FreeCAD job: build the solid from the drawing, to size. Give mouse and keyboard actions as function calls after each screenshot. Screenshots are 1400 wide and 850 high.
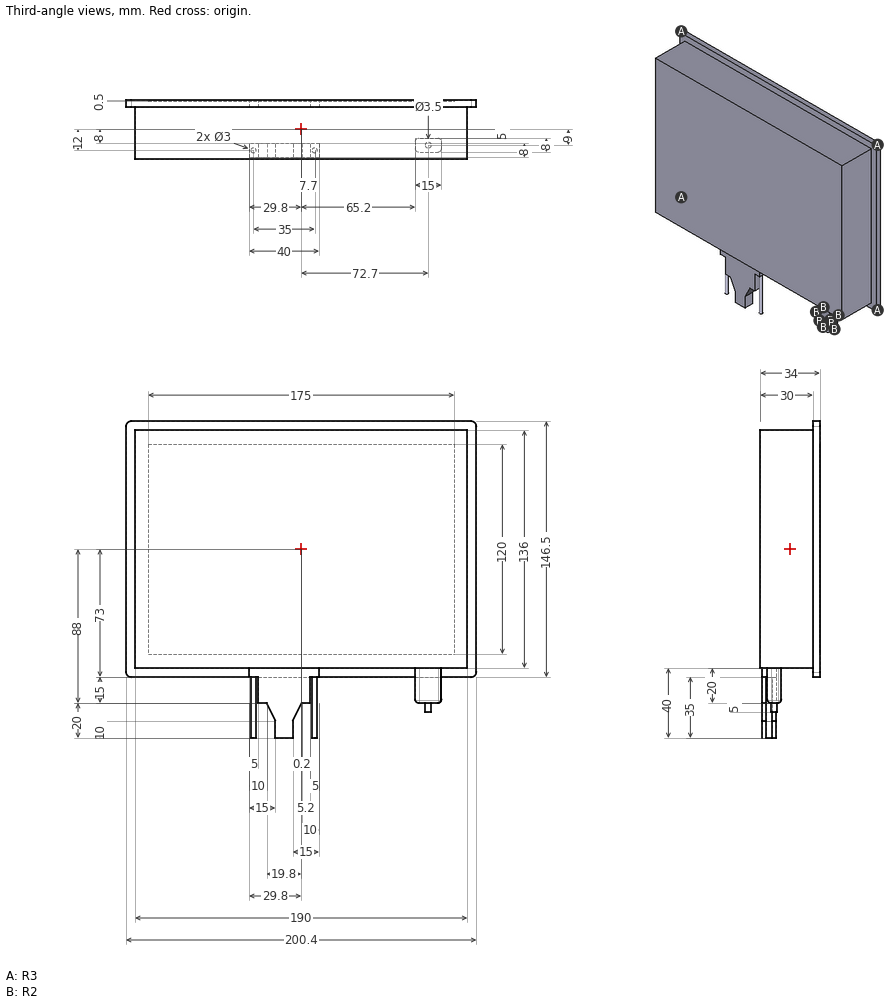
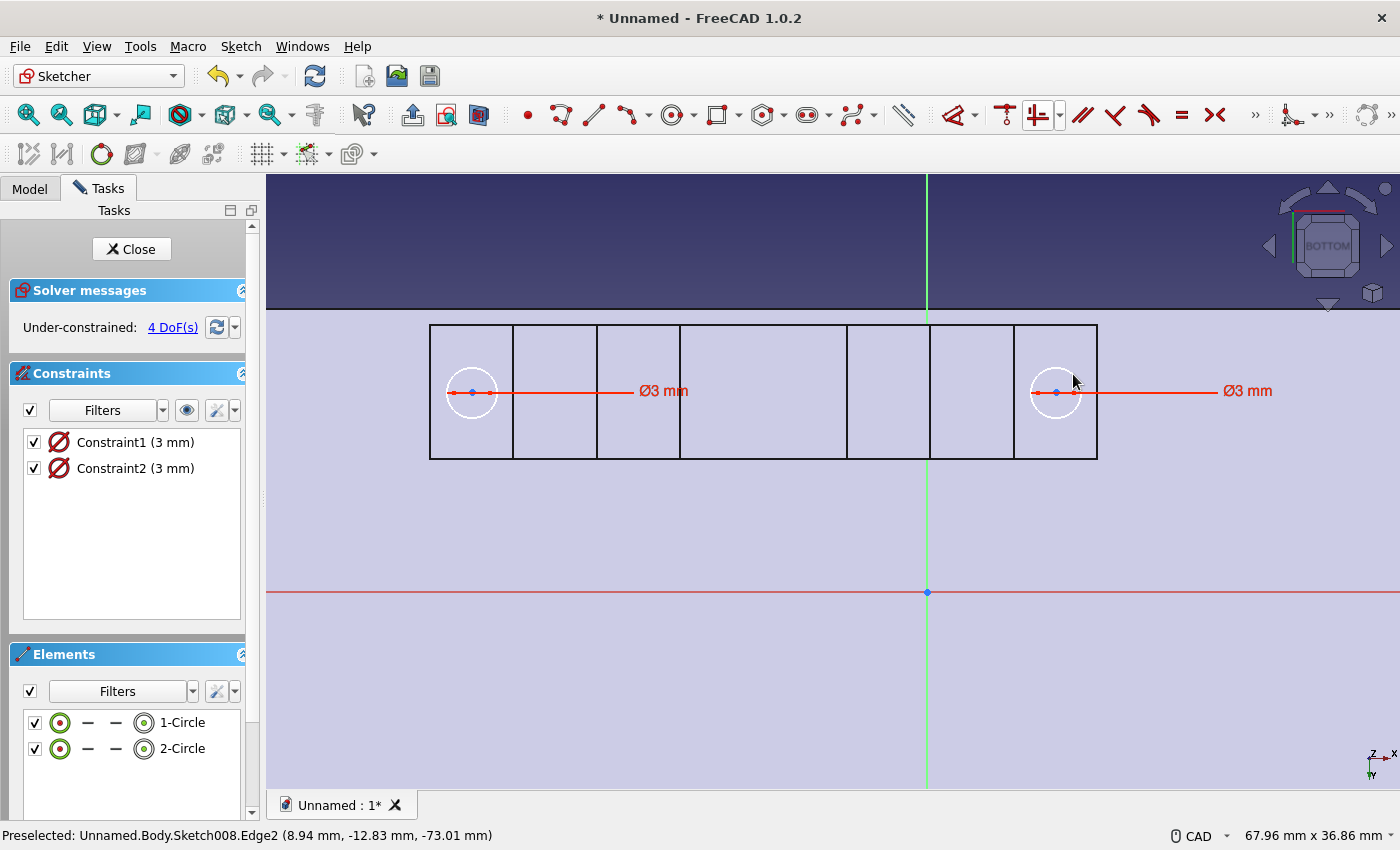
click(952, 116)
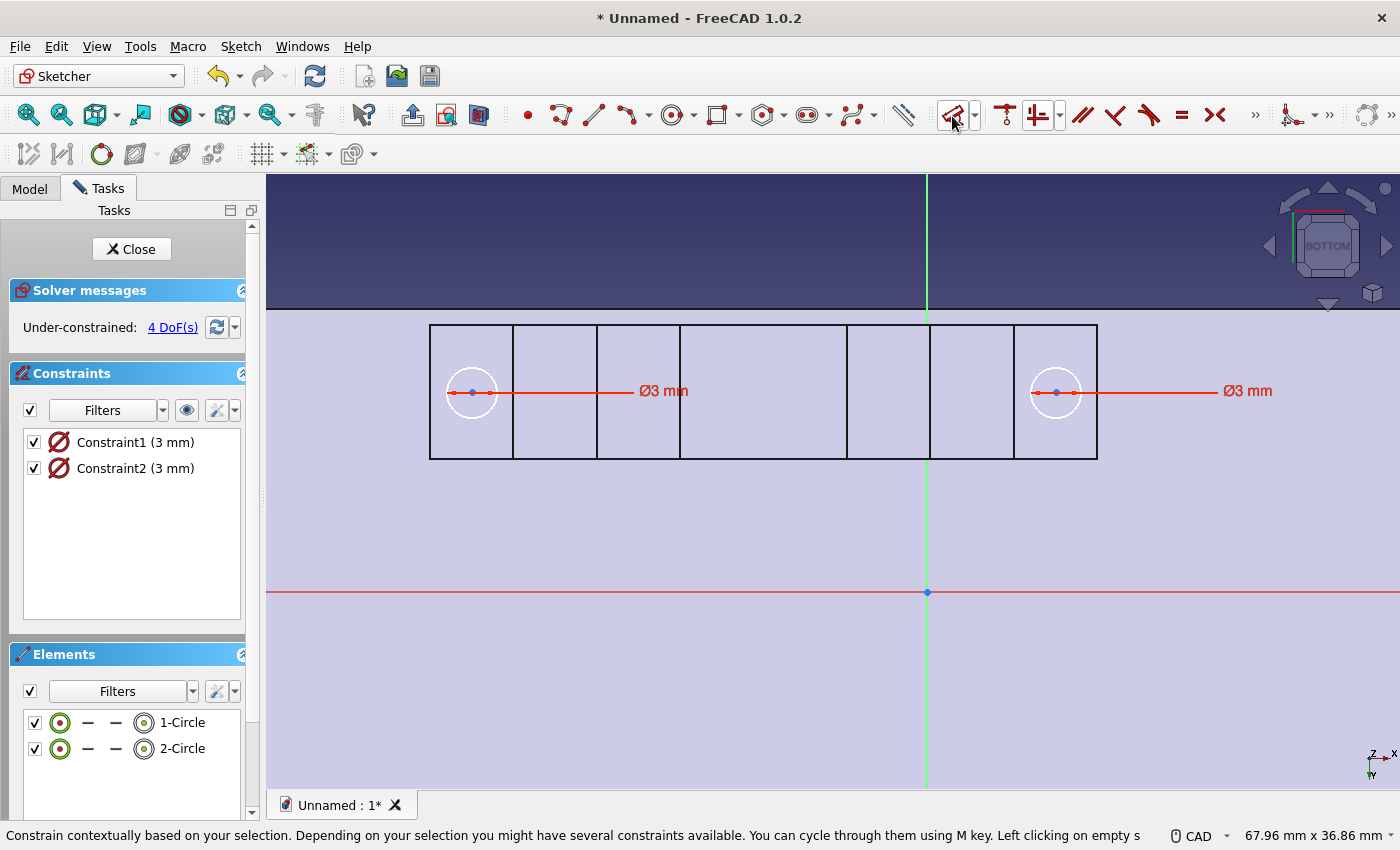
click(472, 393)
click(438, 493)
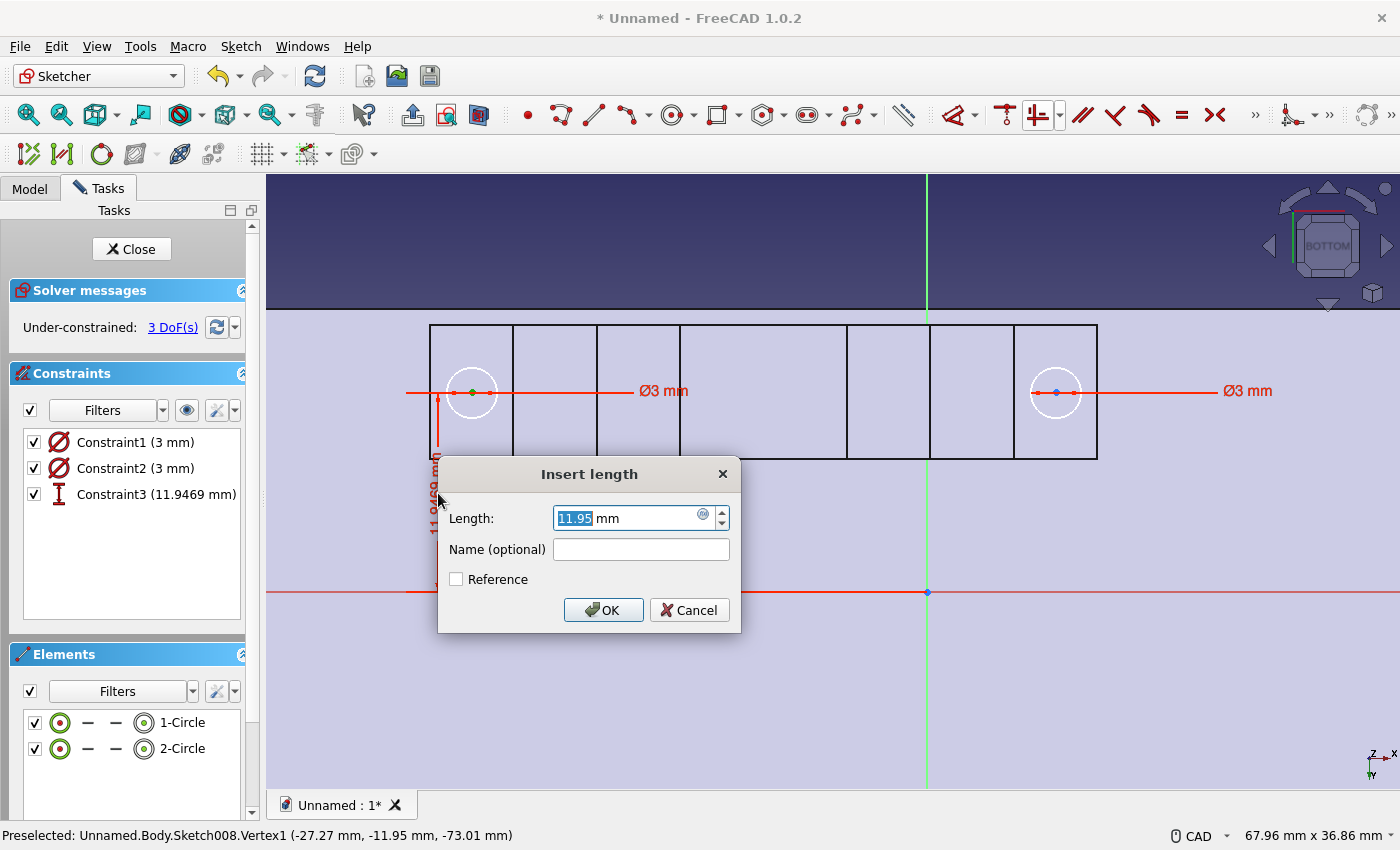
text(12)
key(Return)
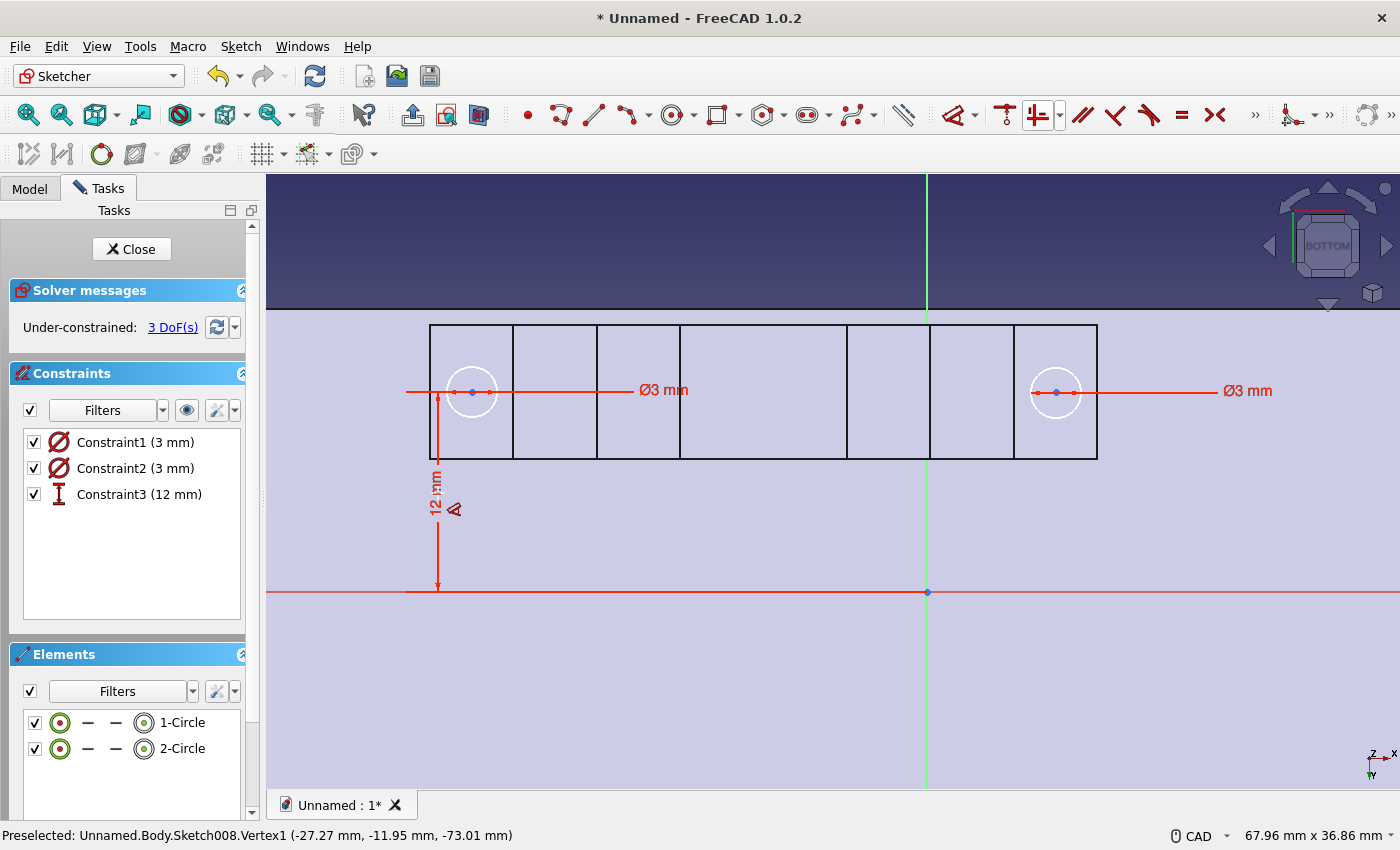
click(1056, 393)
click(1090, 493)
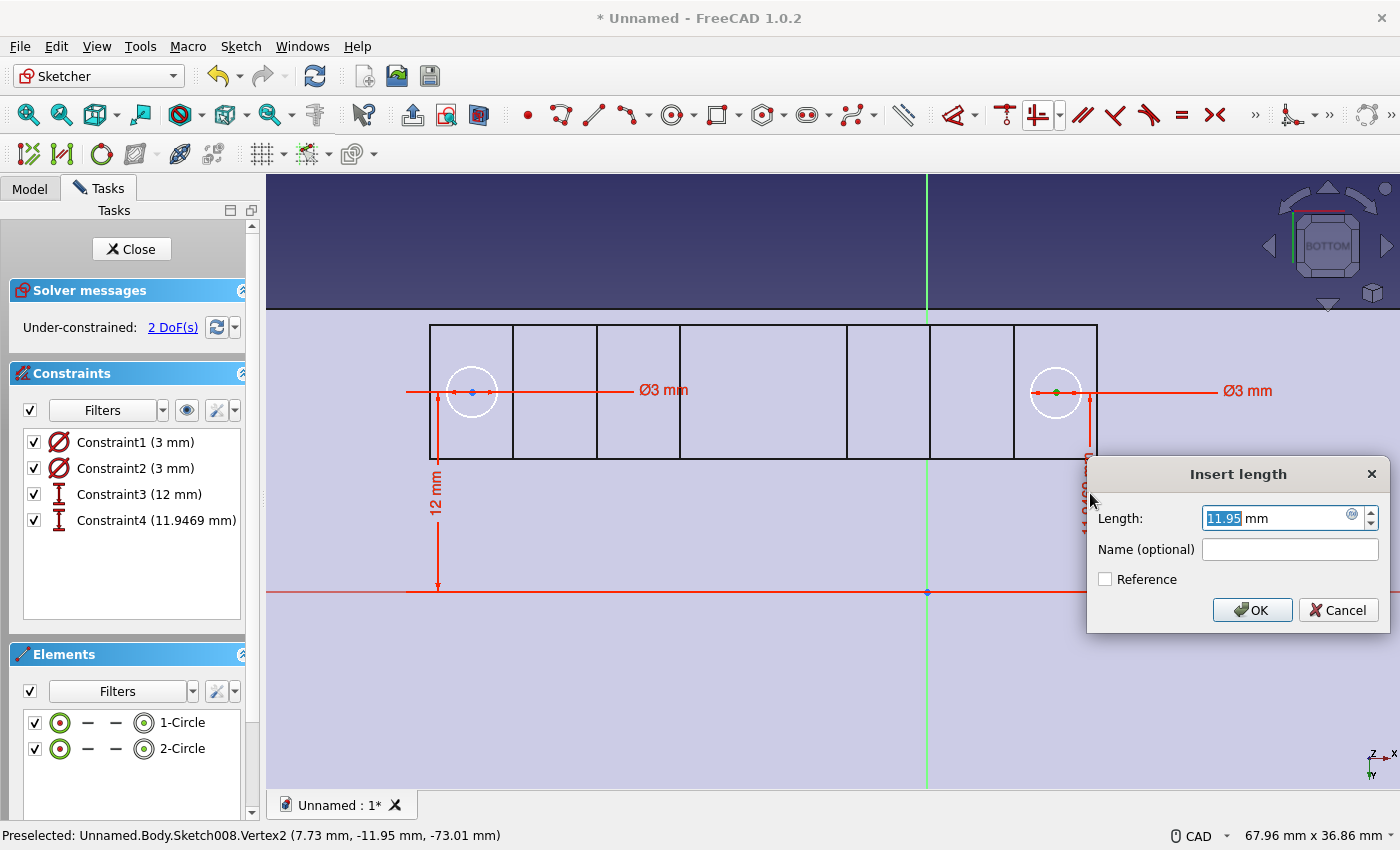
text(12)
key(Return)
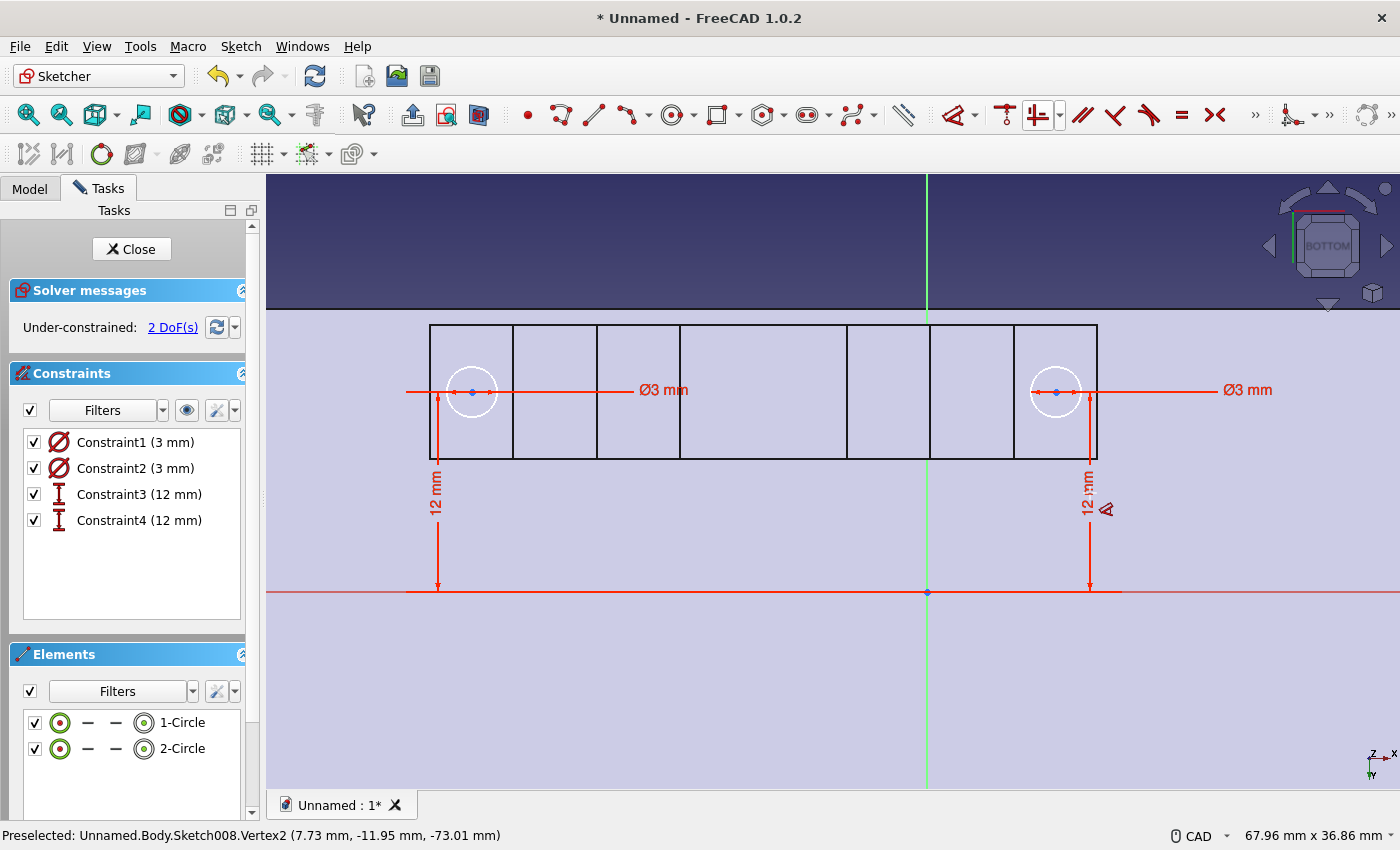
click(1056, 392)
click(992, 626)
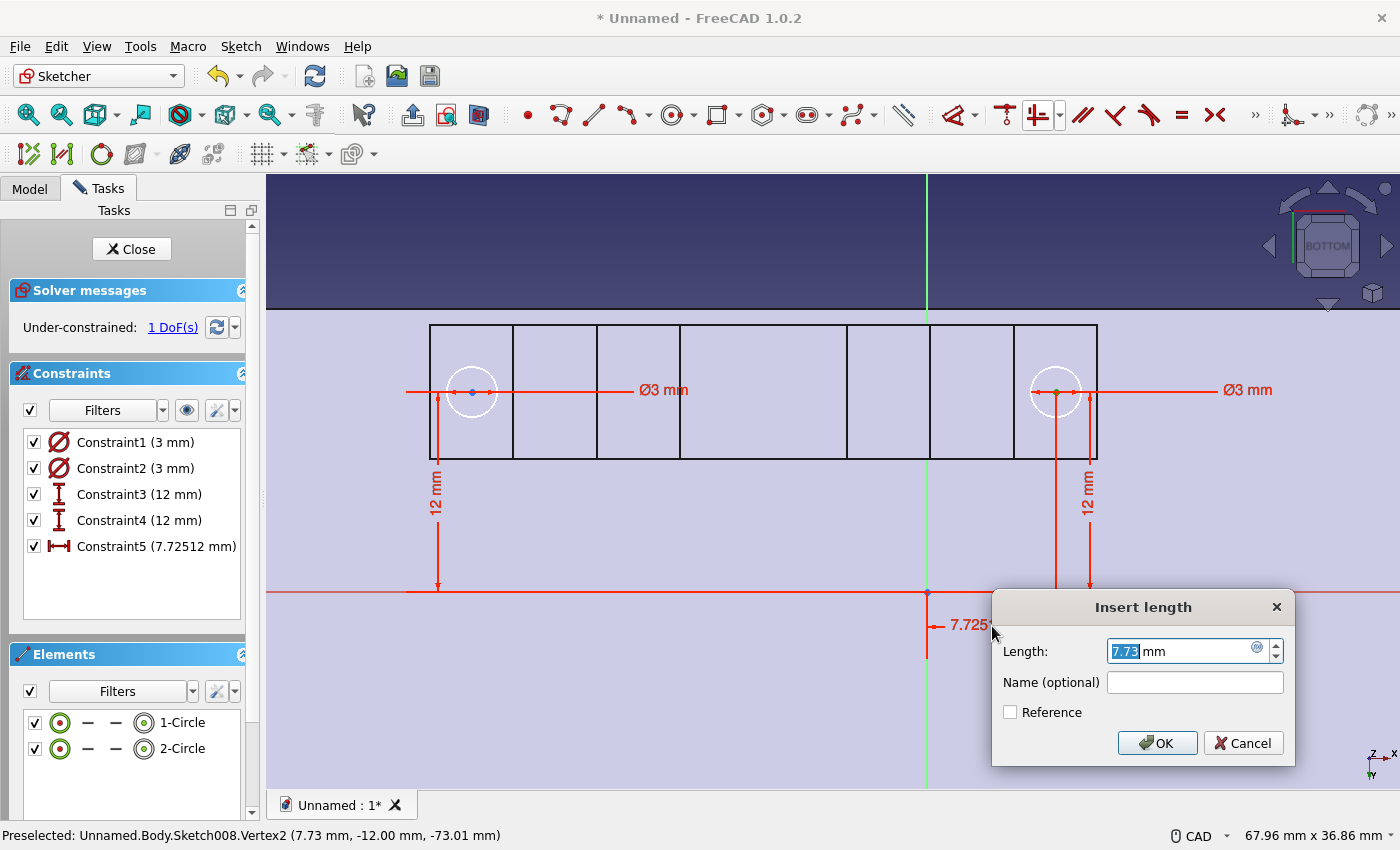
text(7.7)
key(Return)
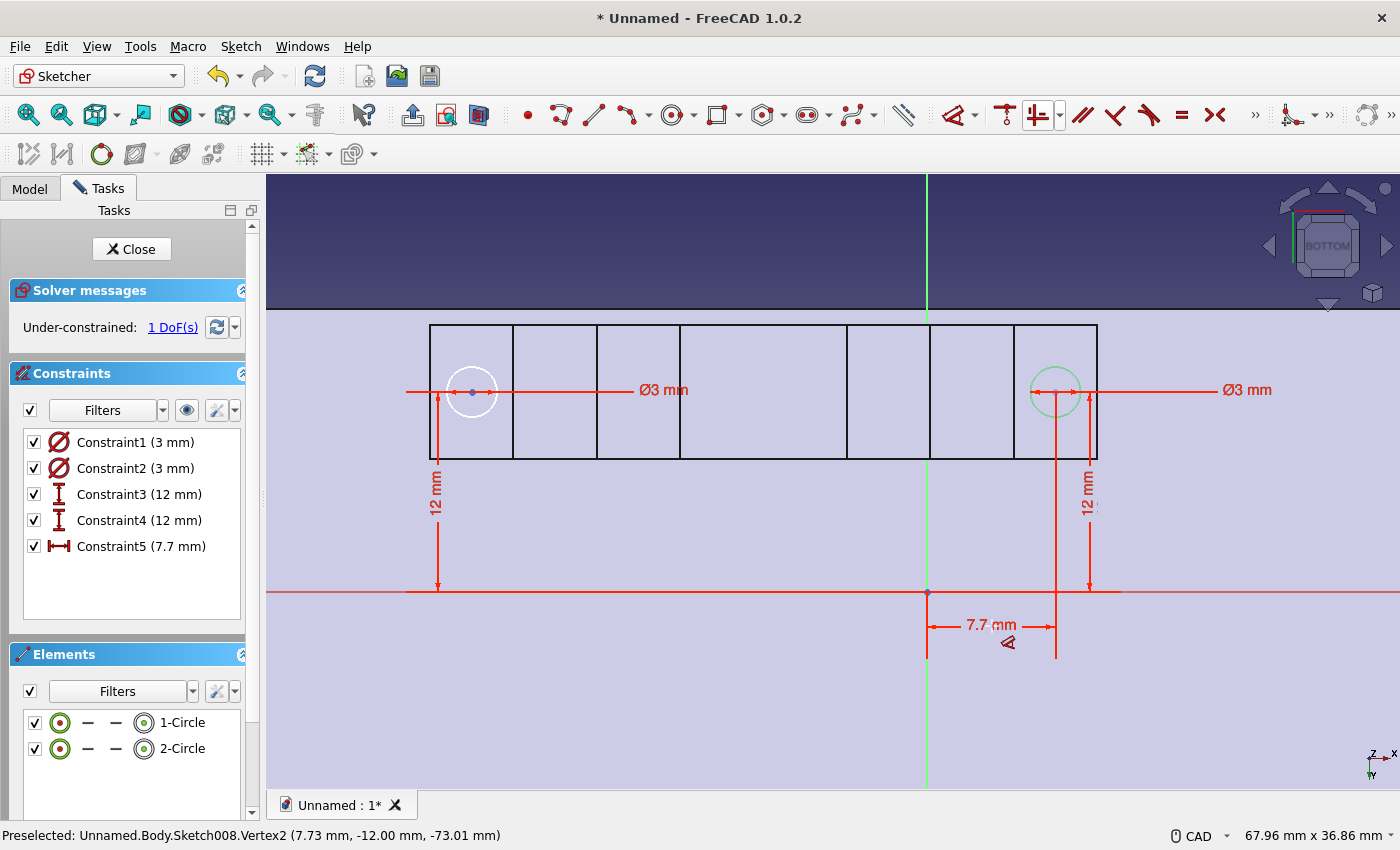
click(472, 392)